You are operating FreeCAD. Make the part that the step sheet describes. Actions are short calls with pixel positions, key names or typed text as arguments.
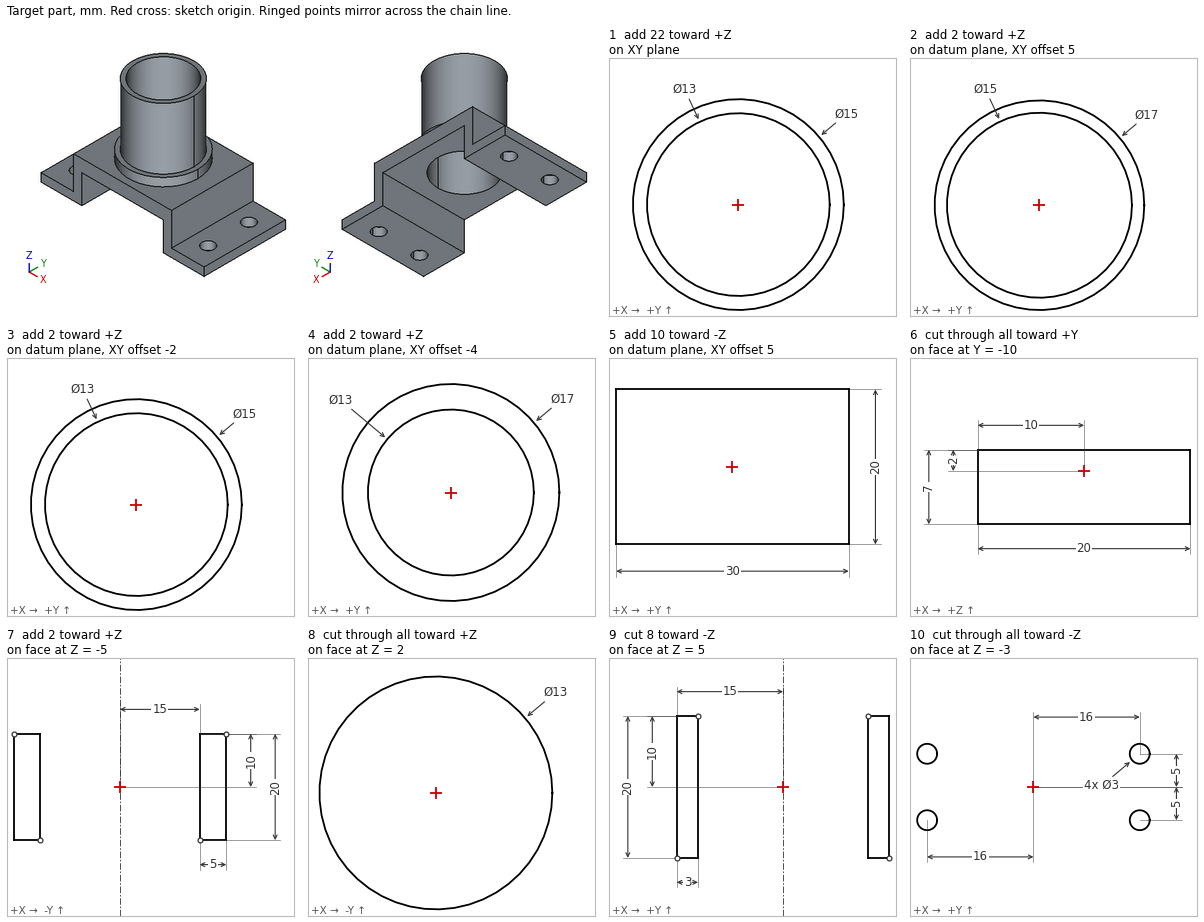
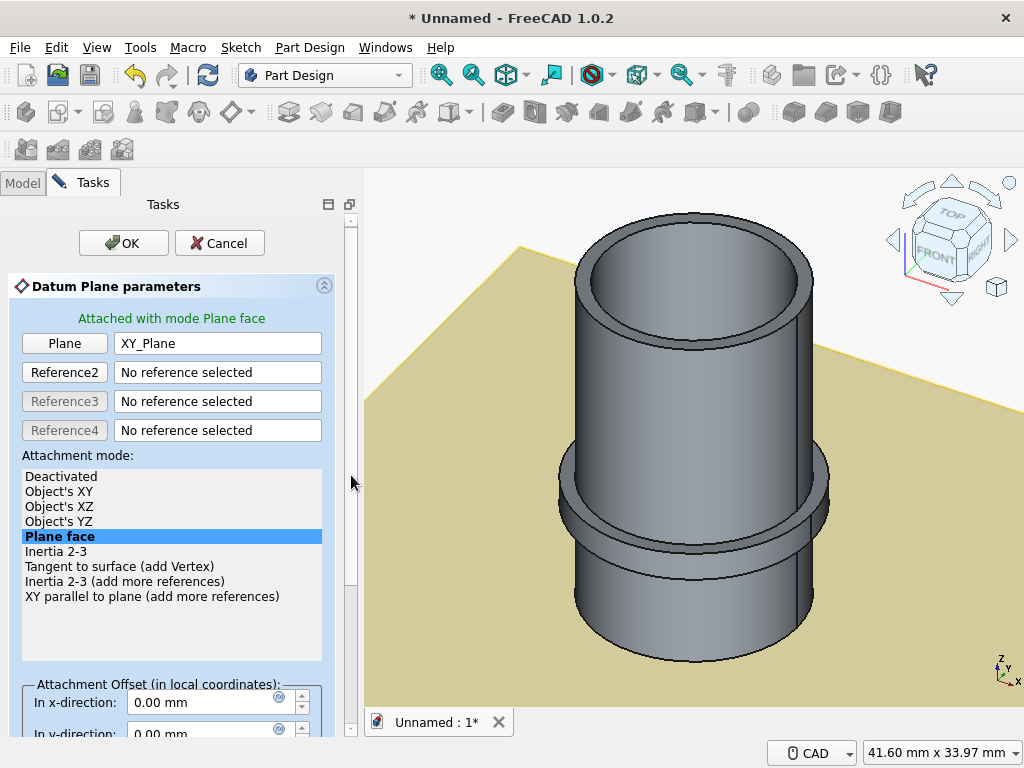
click(124, 243)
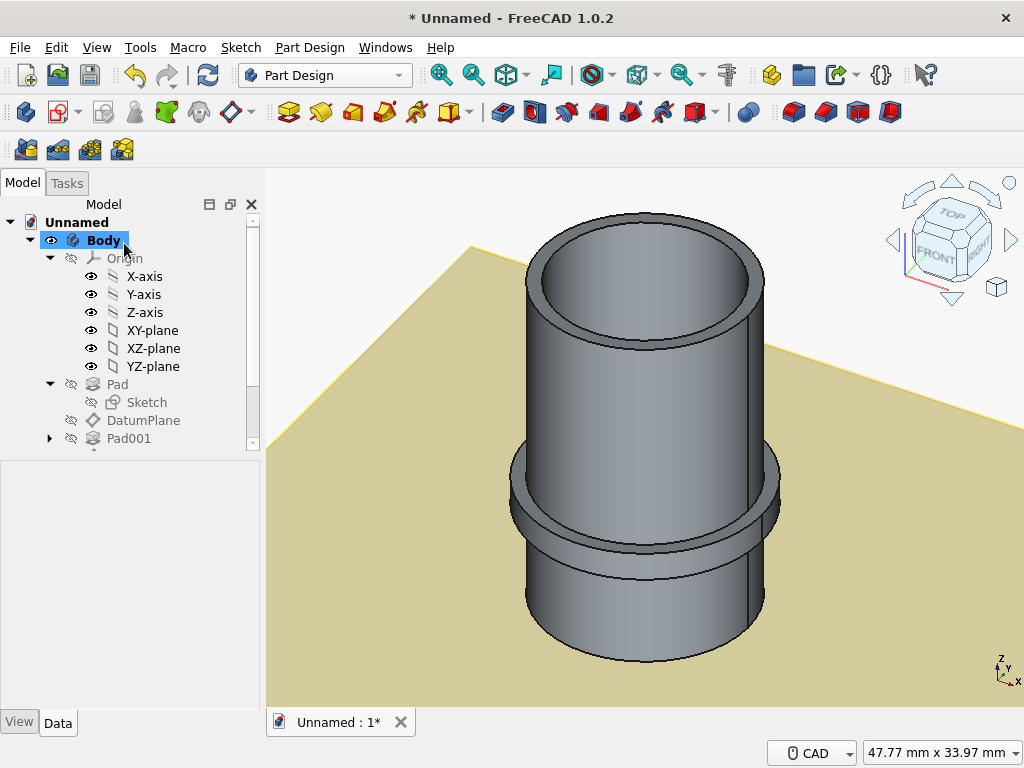
scroll(100, 326, down, 3)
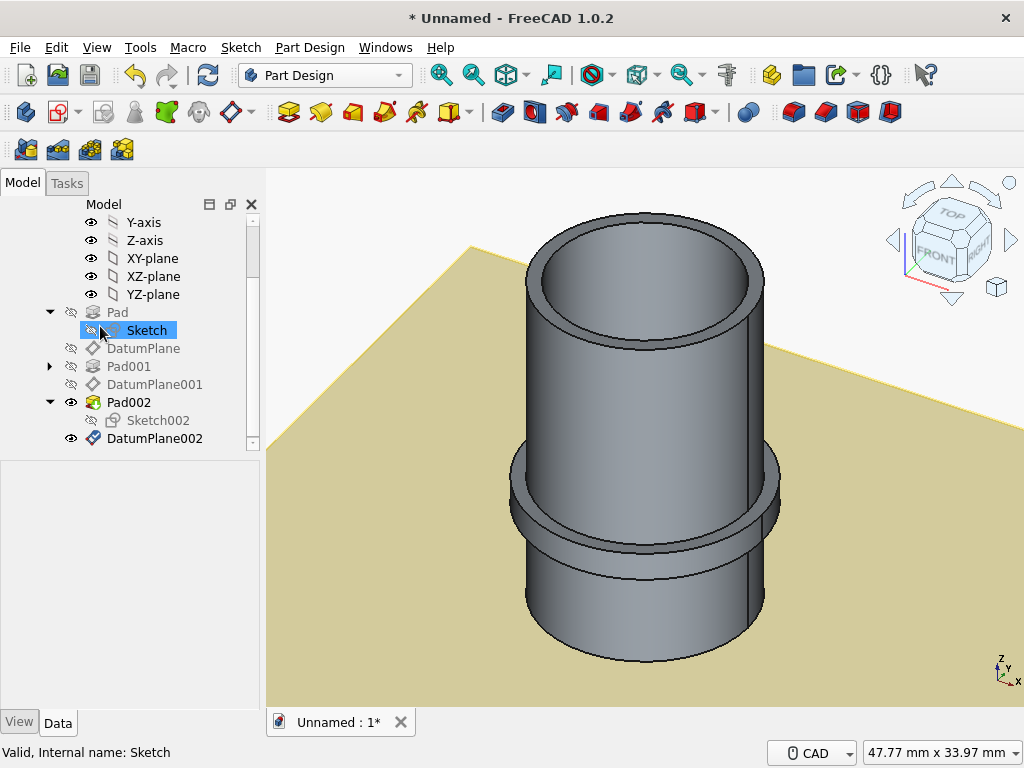
click(116, 438)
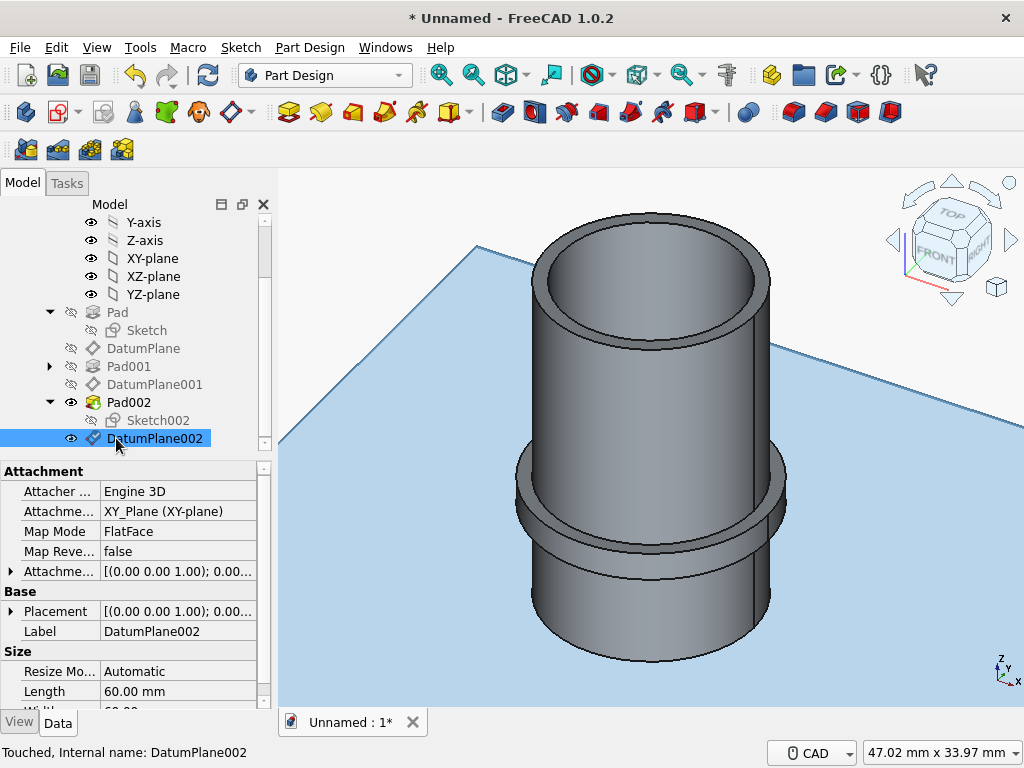
click(58, 112)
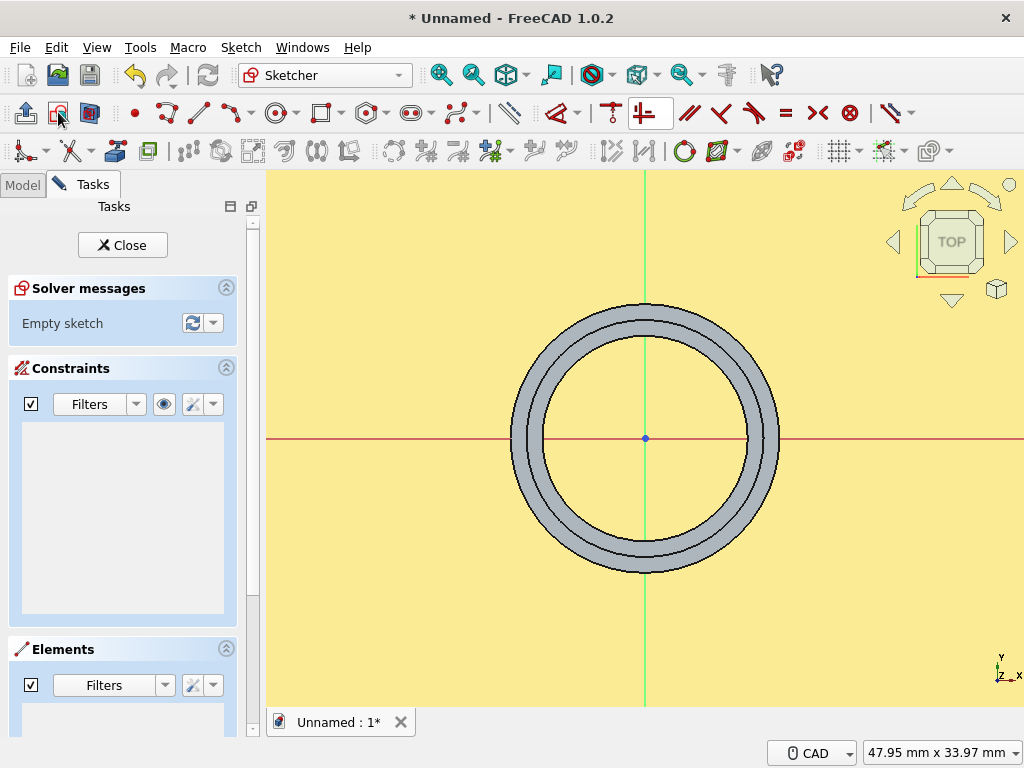
click(90, 114)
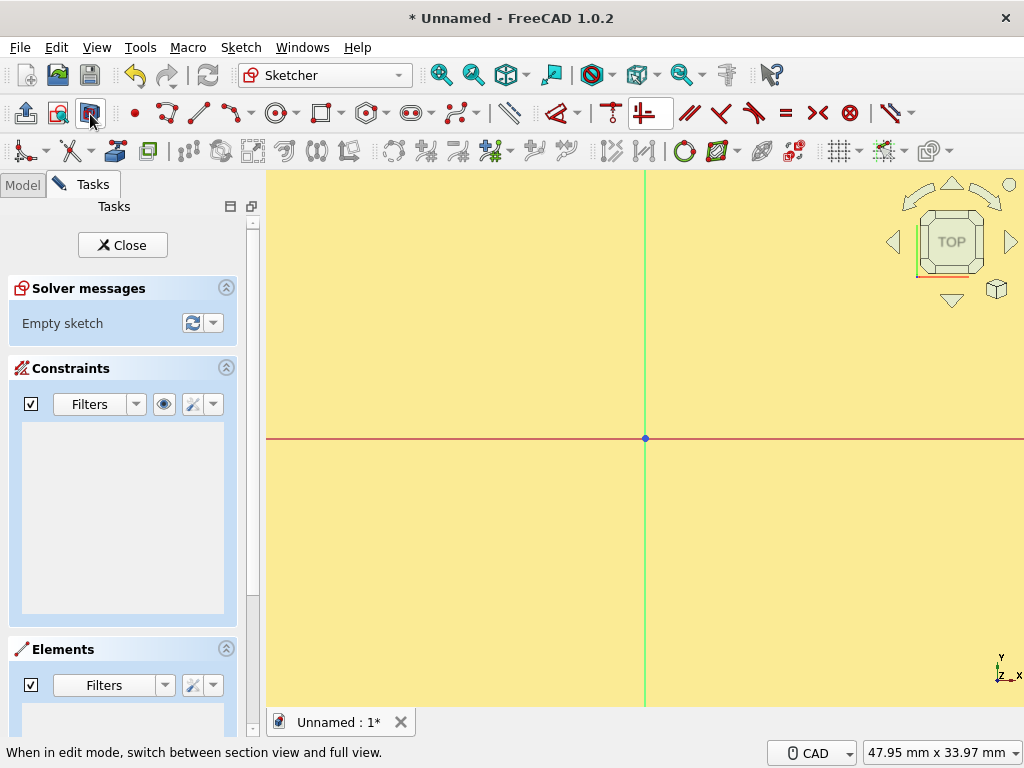
click(276, 114)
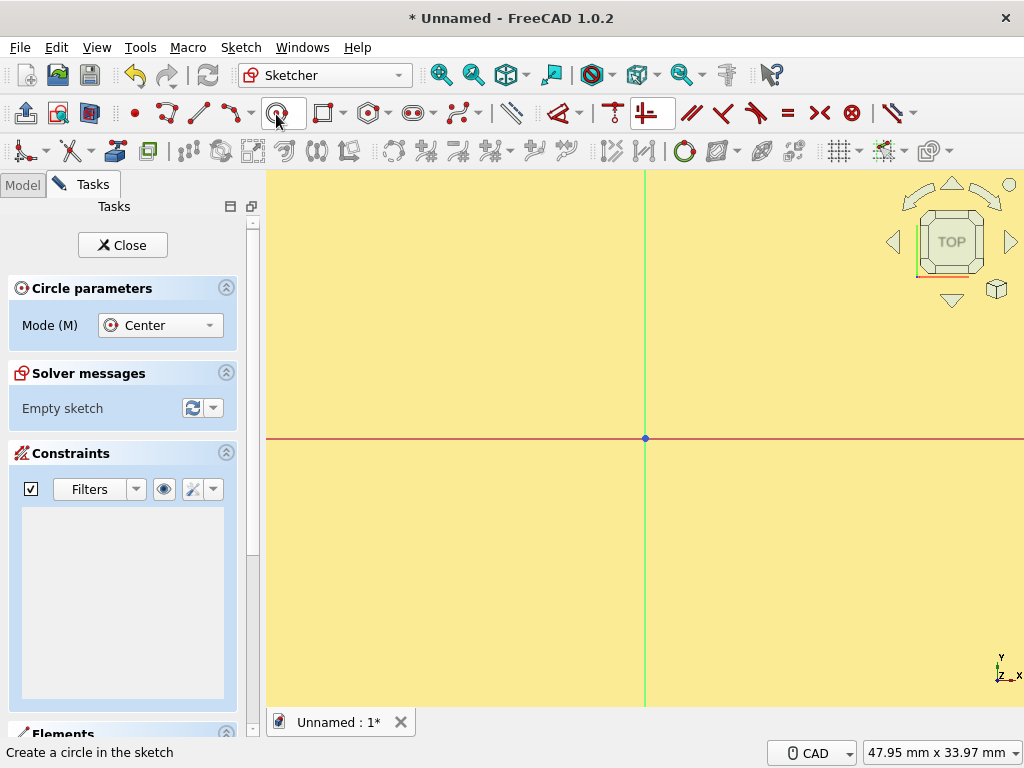
click(645, 438)
click(740, 343)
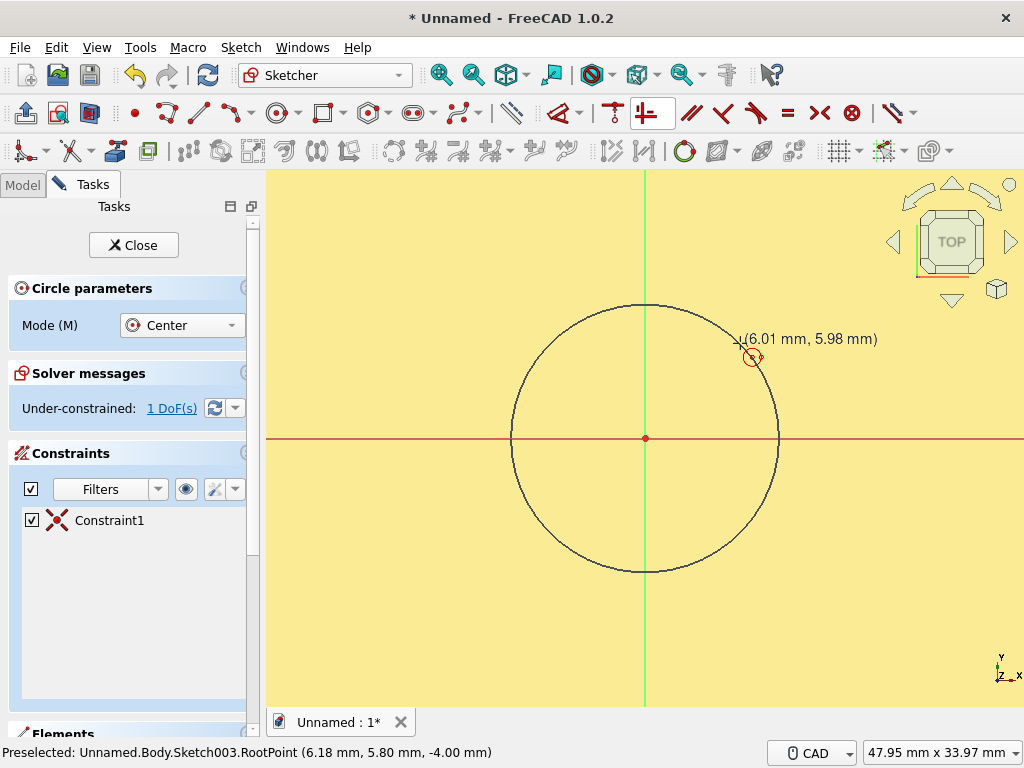
click(645, 438)
click(718, 366)
key(Escape)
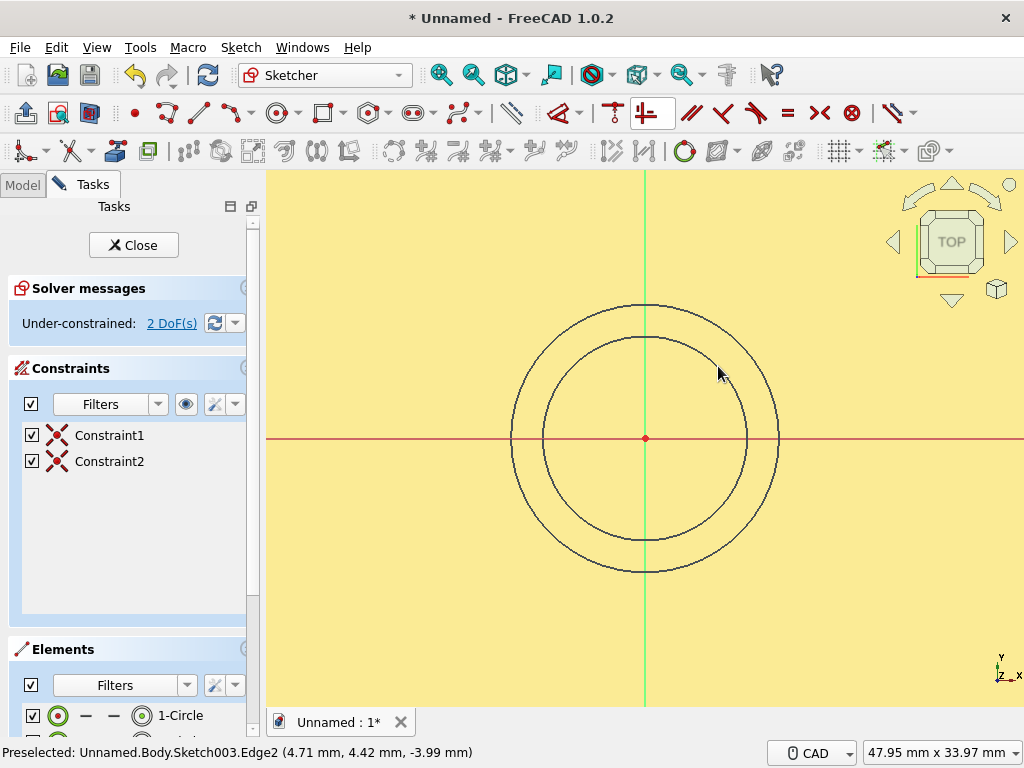
click(558, 114)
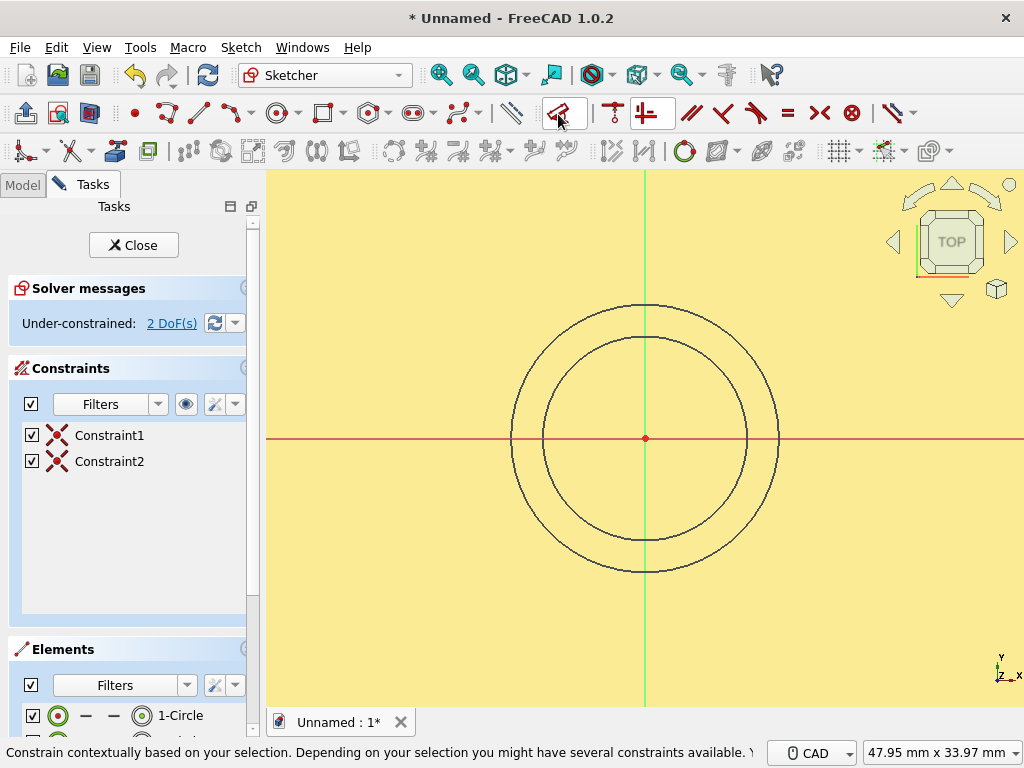
click(739, 343)
click(761, 320)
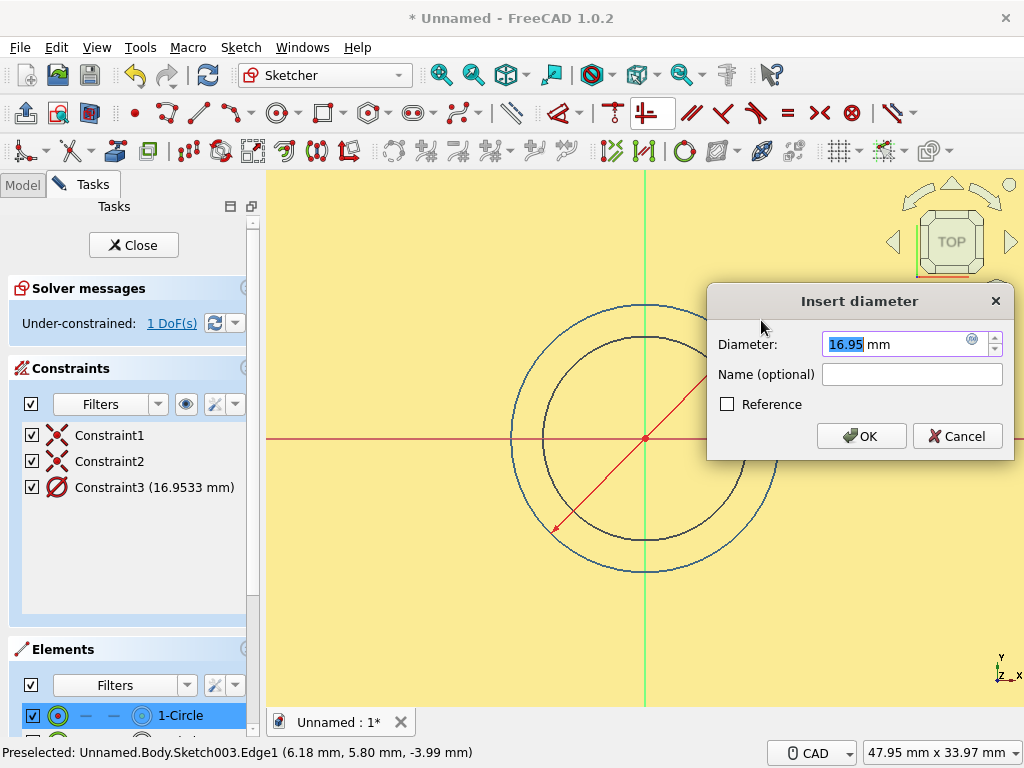
text(17)
key(Return)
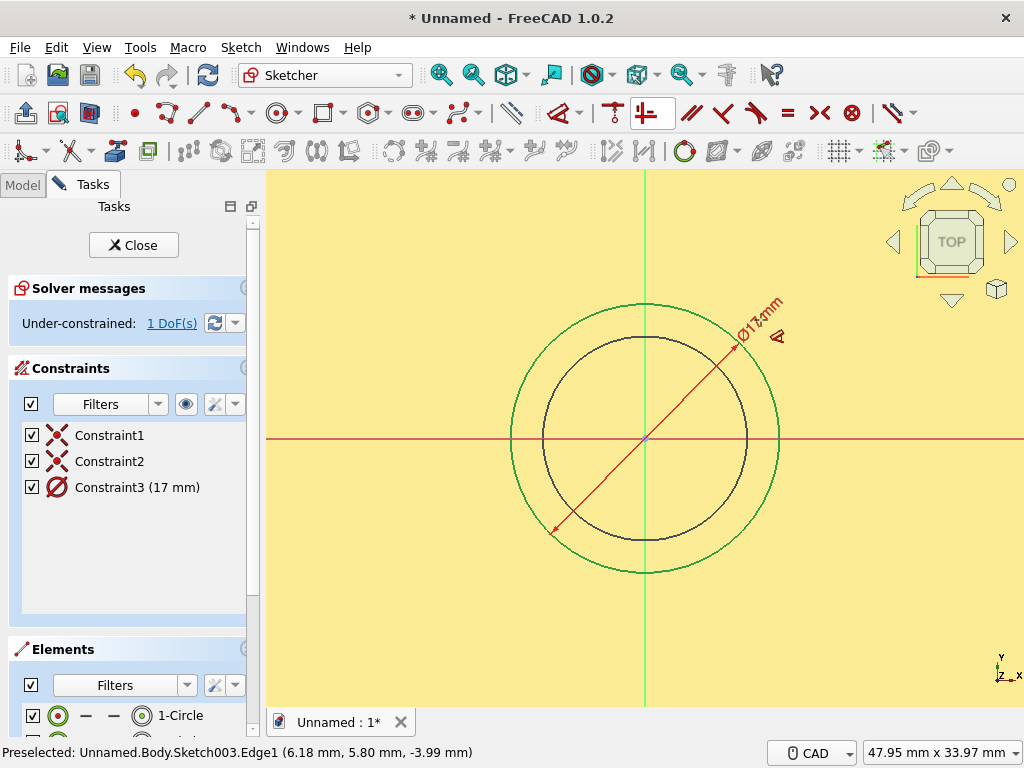
click(717, 366)
click(796, 394)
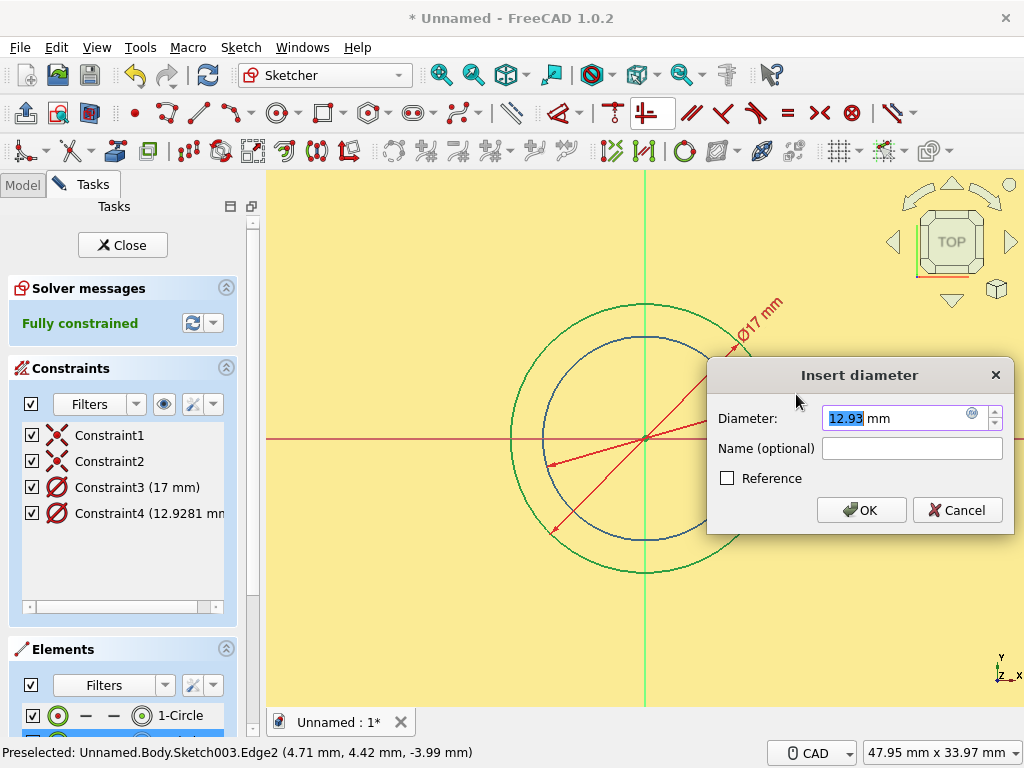
text(13)
key(Return)
key(Escape)